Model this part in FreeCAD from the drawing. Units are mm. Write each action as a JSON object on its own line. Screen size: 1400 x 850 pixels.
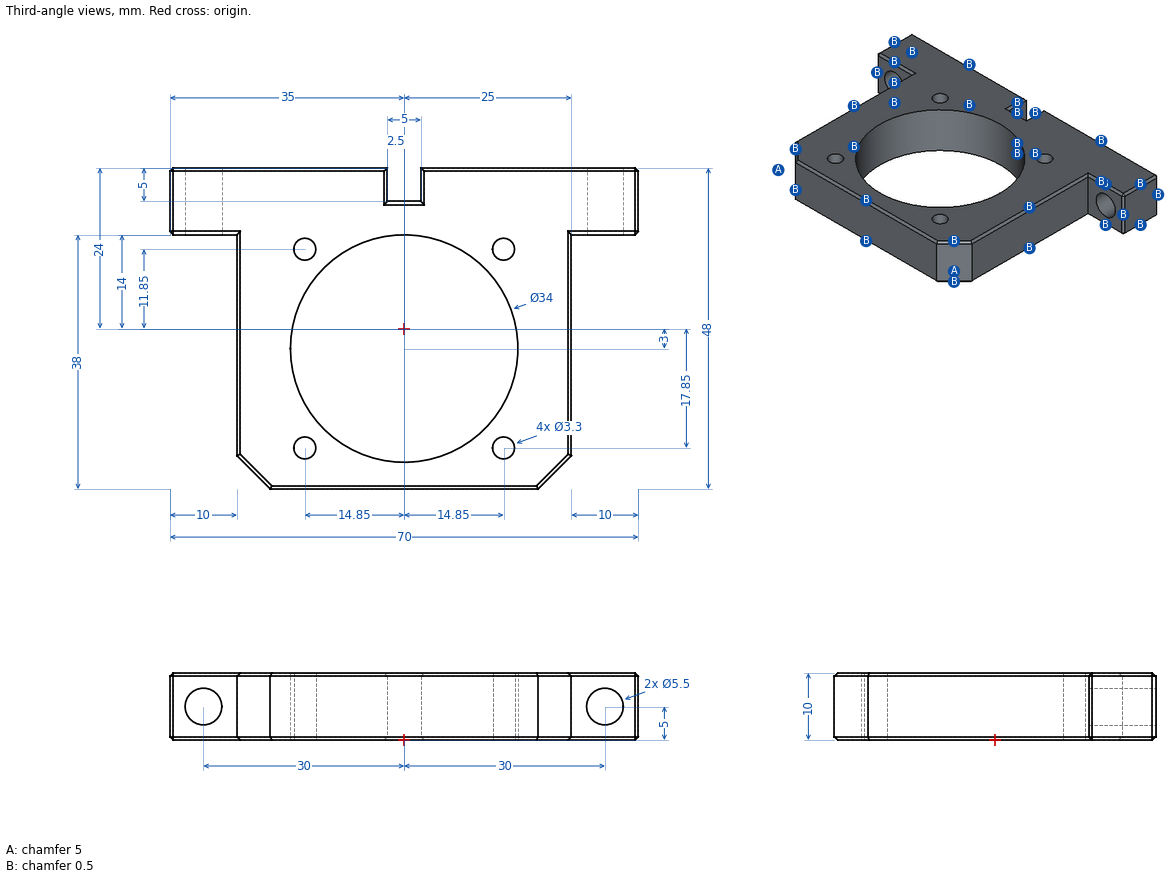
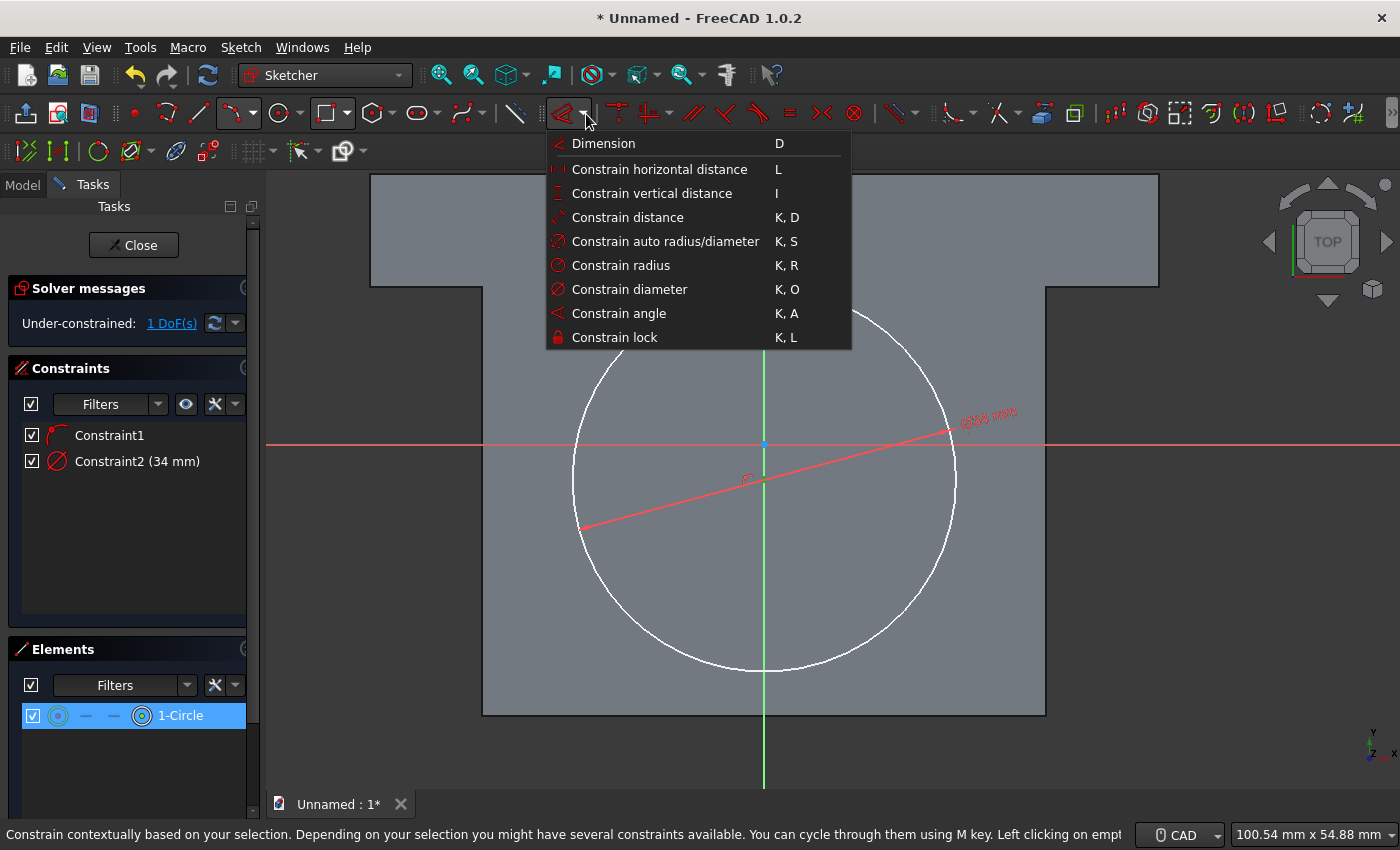
{"action": "left_click", "coordinate": [699, 193]}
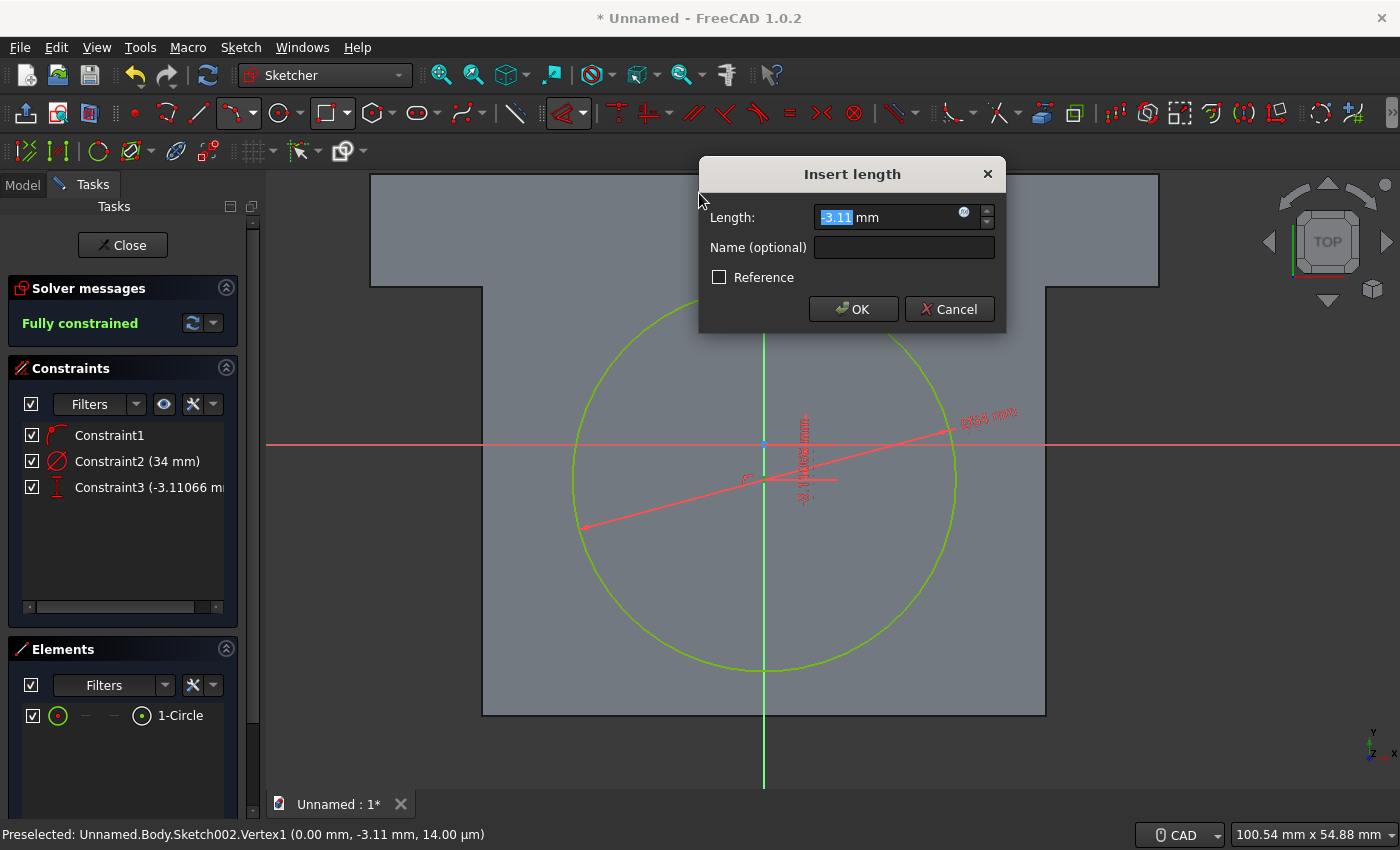
{"action": "type", "text": "-3"}
{"action": "key", "text": "Return"}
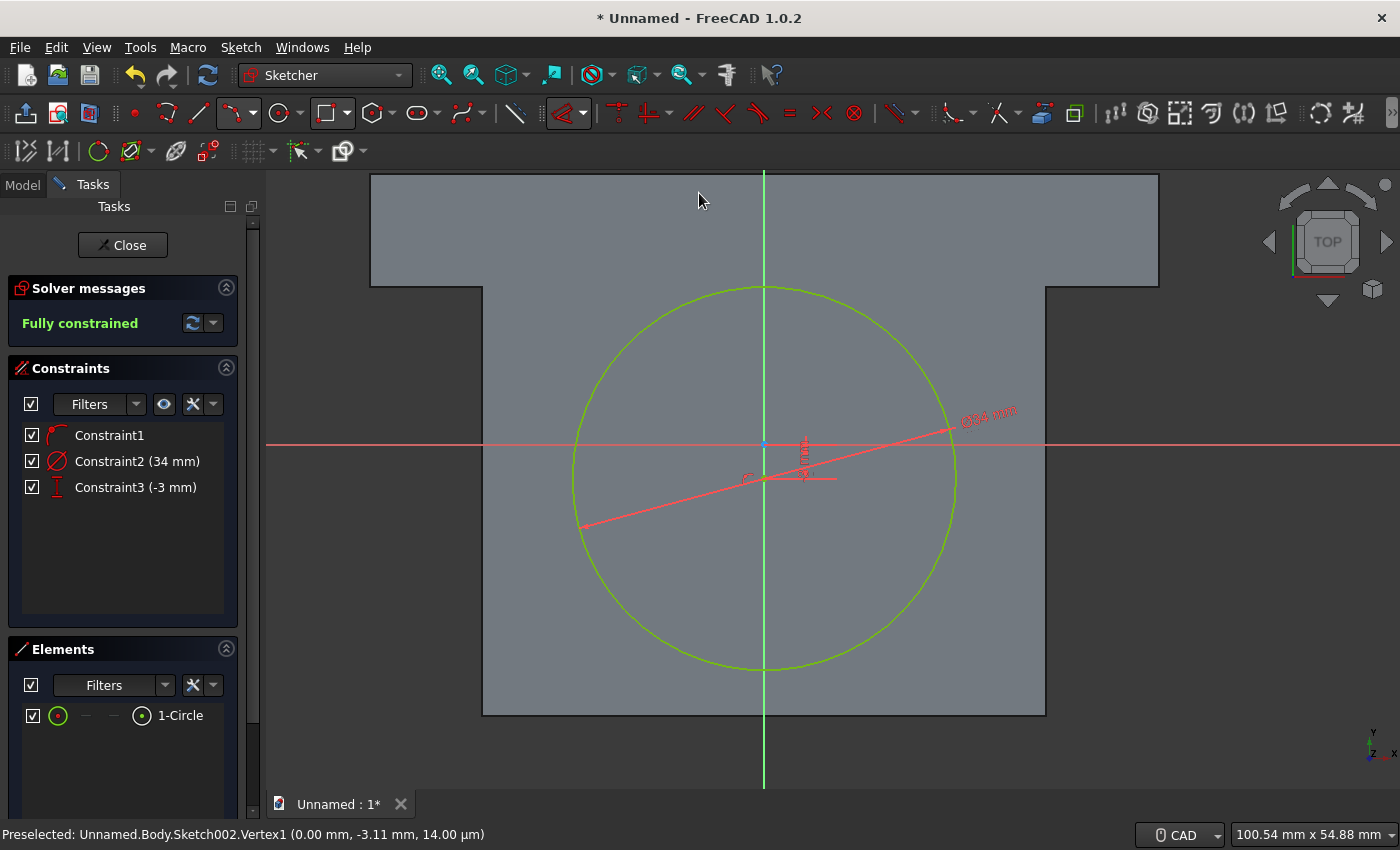
{"action": "left_click", "coordinate": [123, 245]}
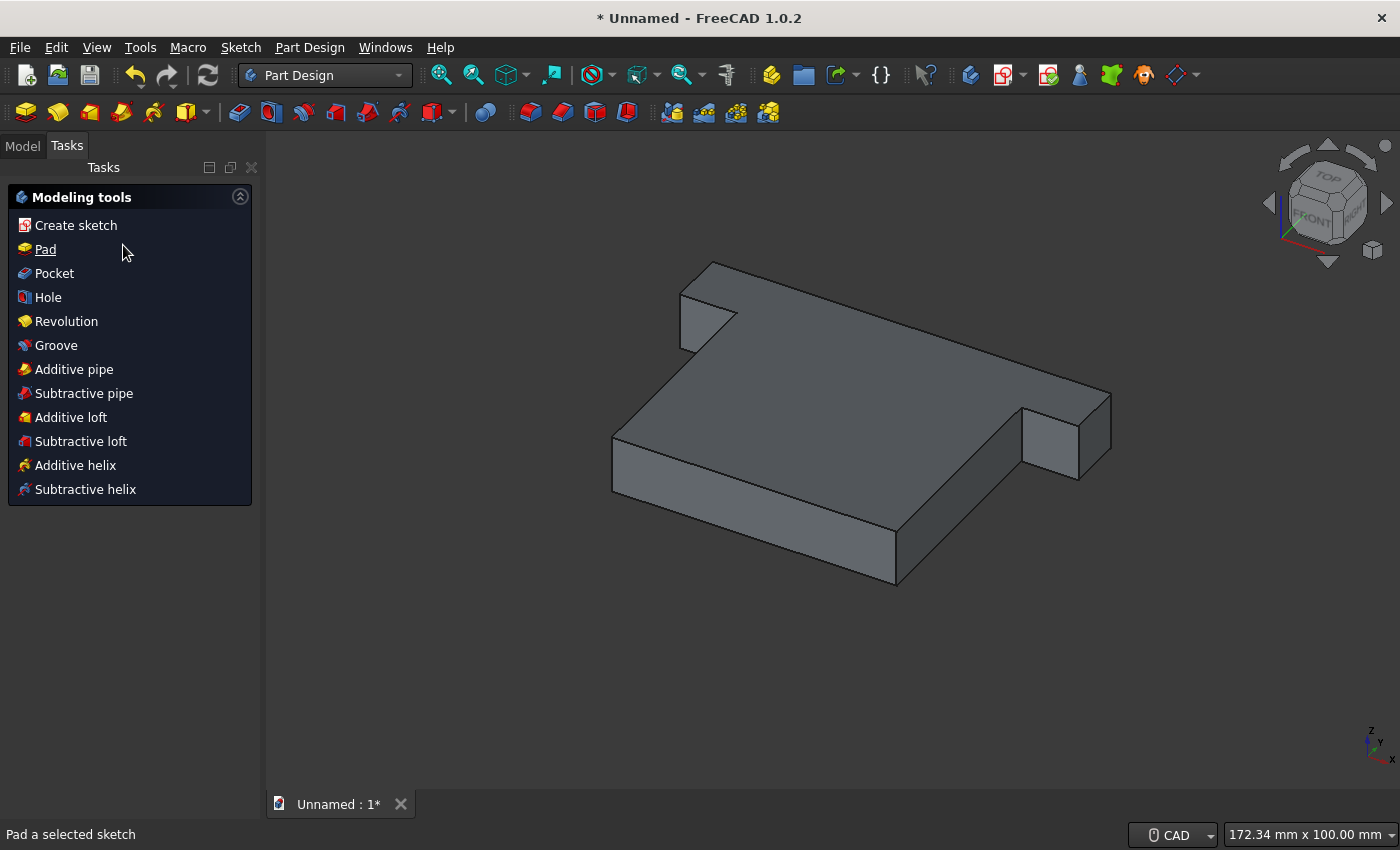
{"action": "left_click", "coordinate": [240, 112]}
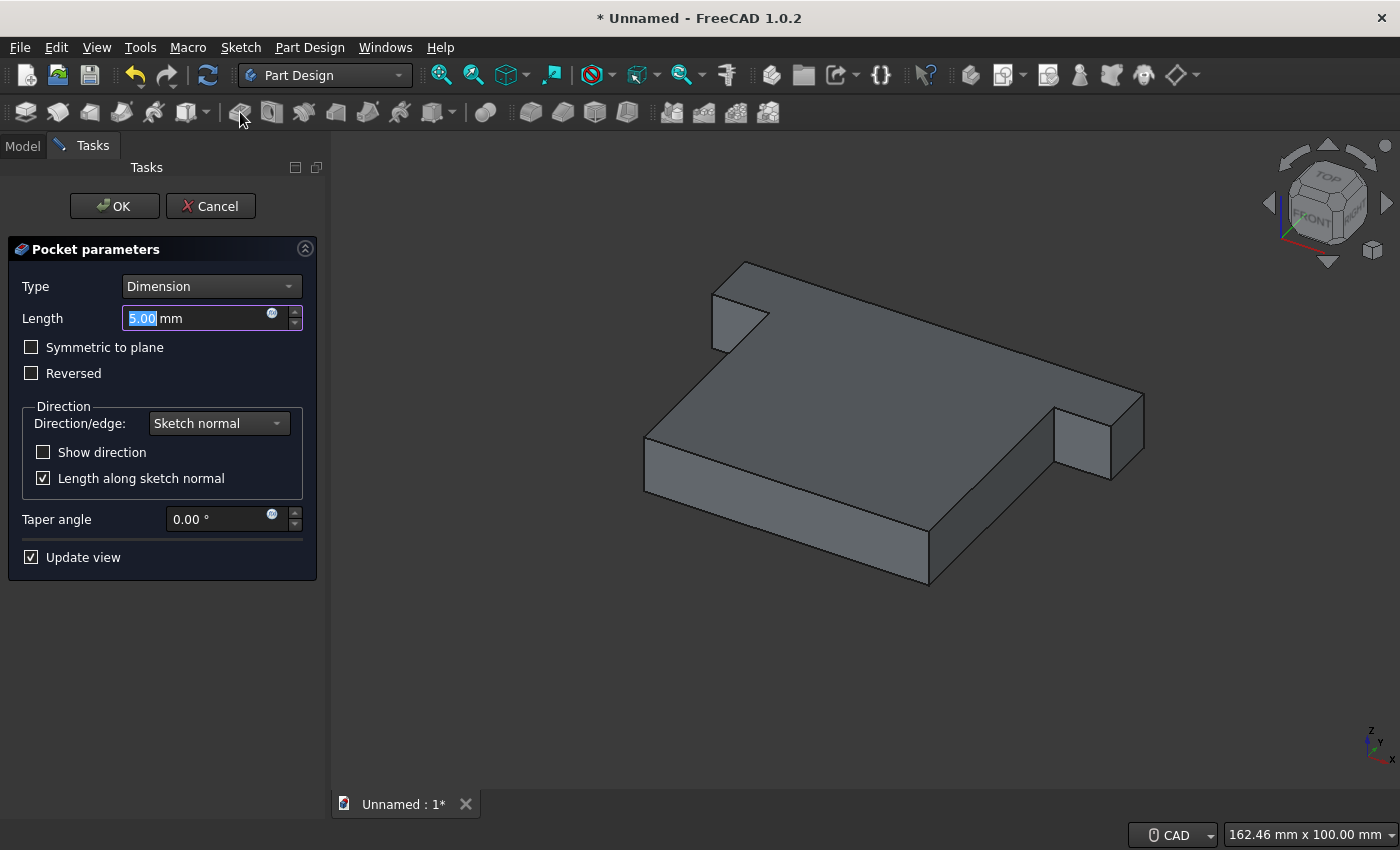
{"action": "left_click", "coordinate": [212, 286]}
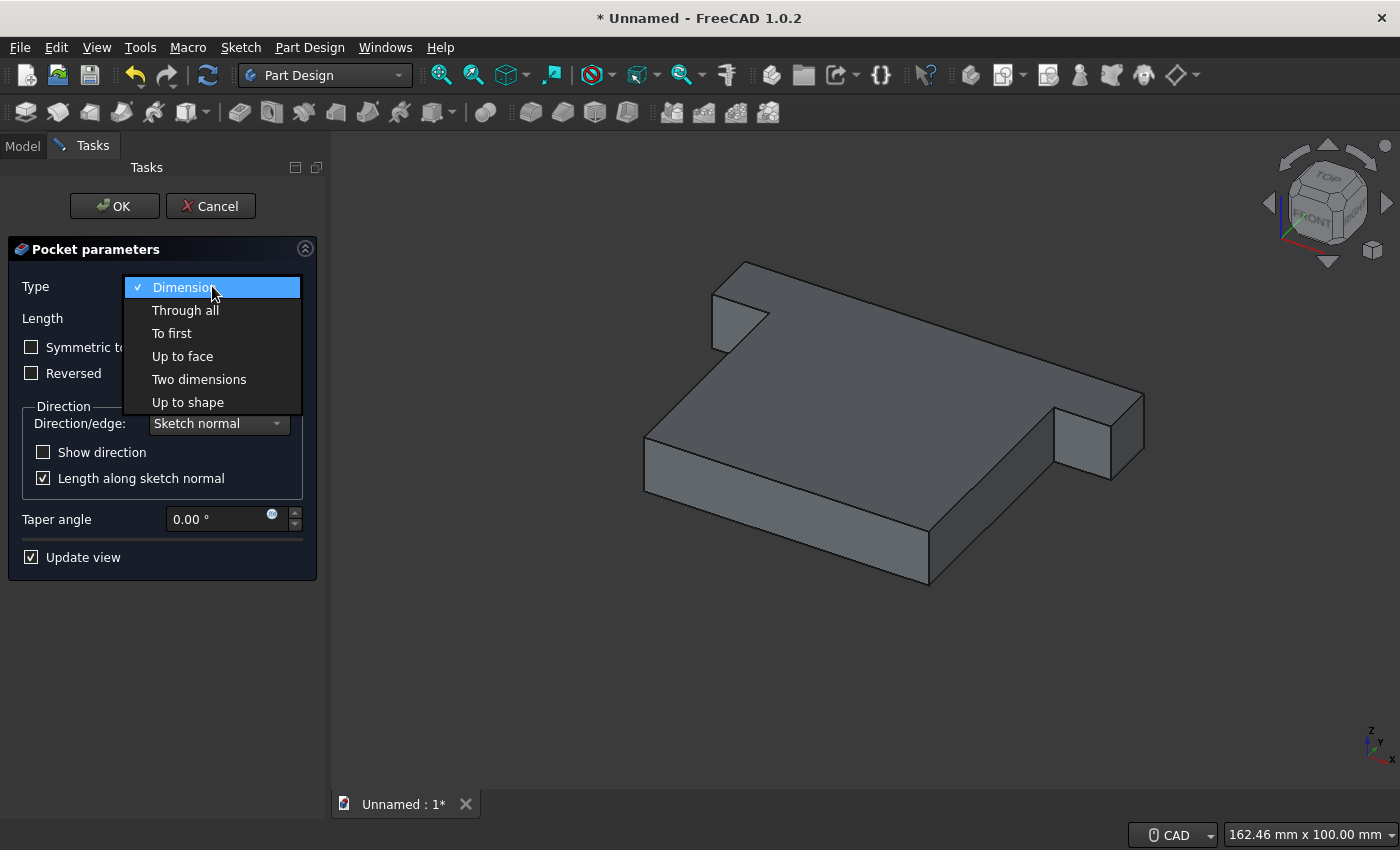
{"action": "left_click", "coordinate": [212, 310]}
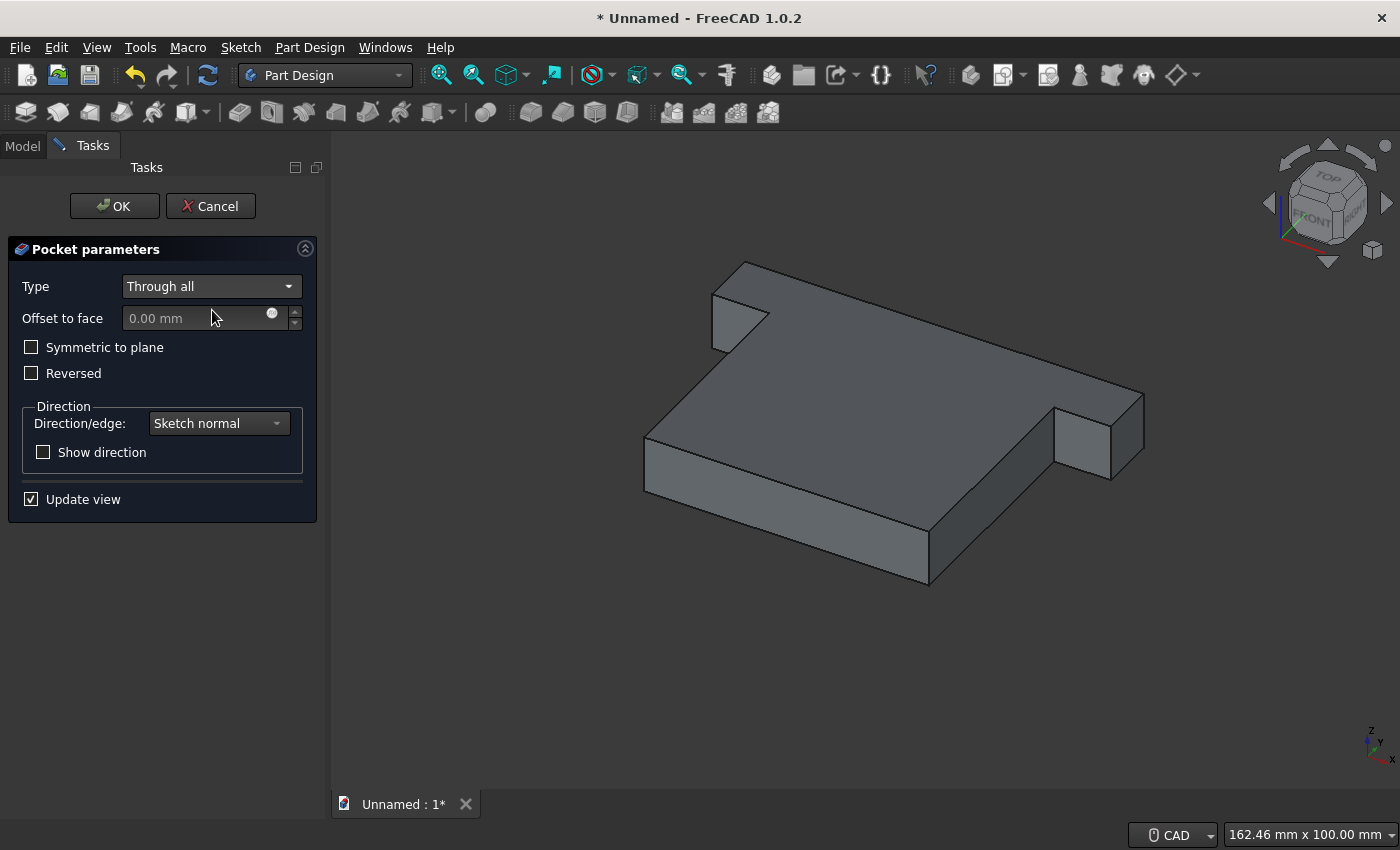
{"action": "left_click", "coordinate": [30, 373]}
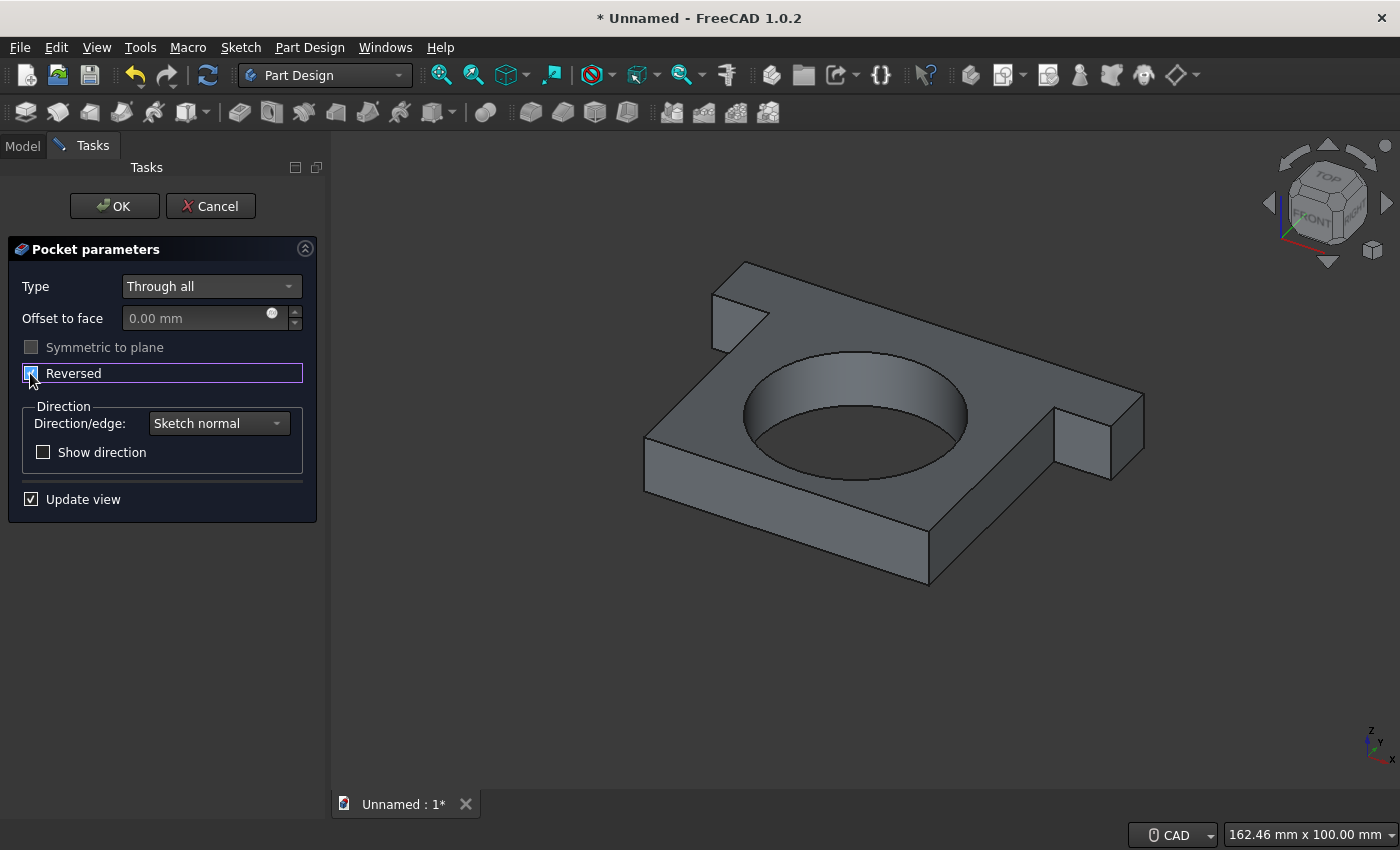
{"action": "left_click", "coordinate": [115, 206]}